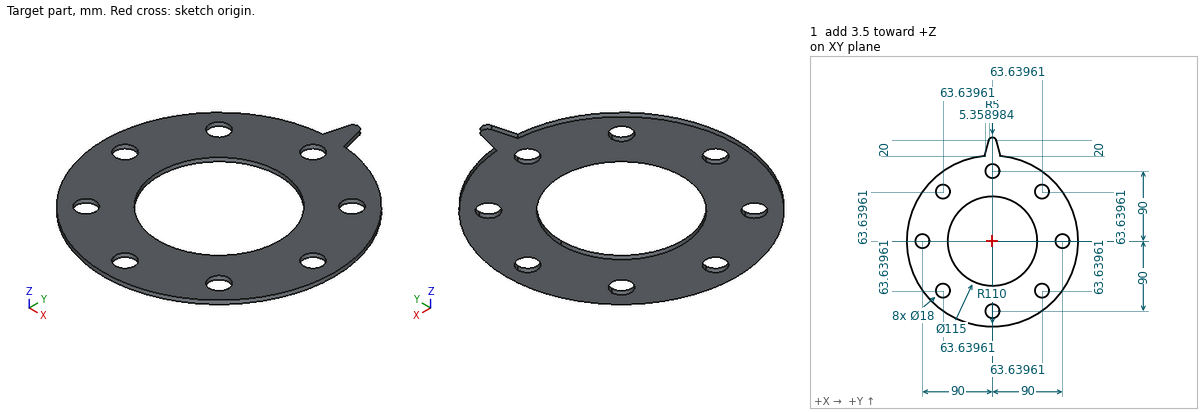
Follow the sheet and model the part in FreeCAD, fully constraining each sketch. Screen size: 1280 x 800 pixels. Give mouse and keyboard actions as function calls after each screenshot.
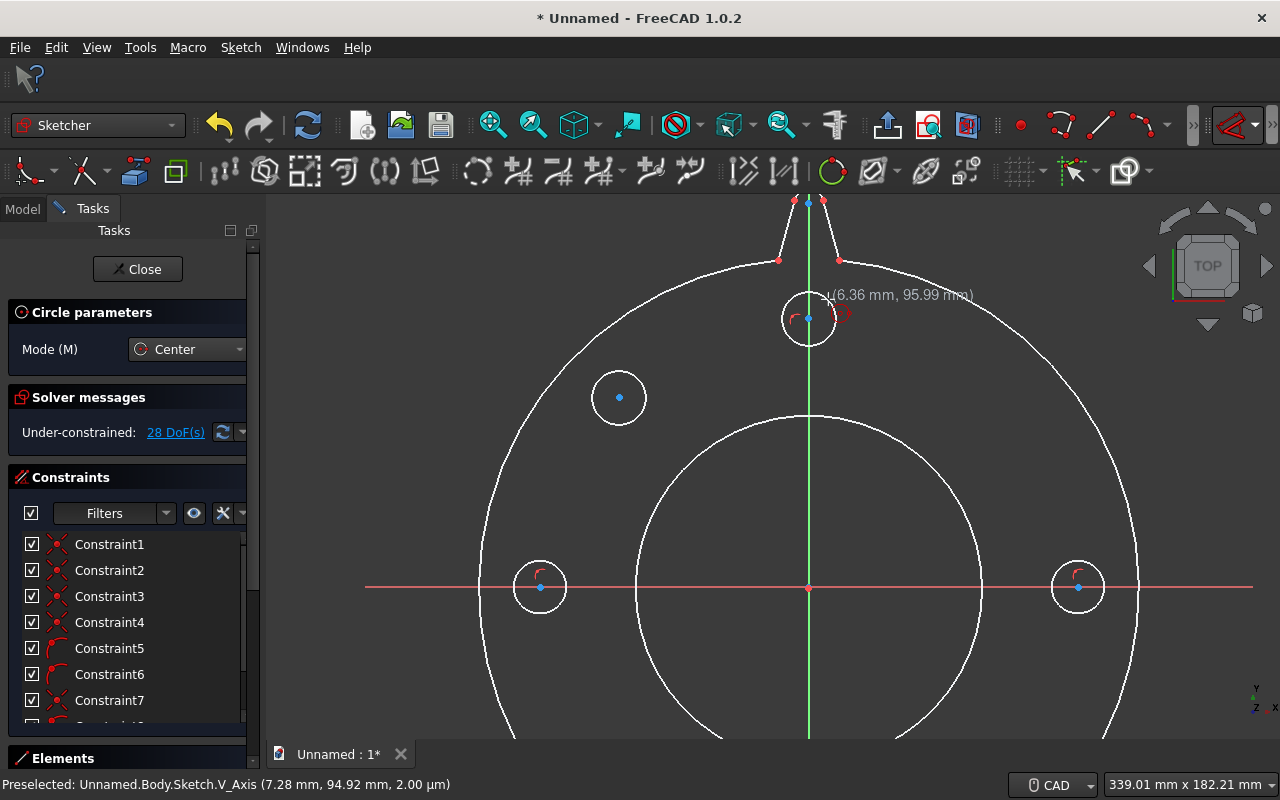
click(999, 397)
click(1018, 378)
key(Escape)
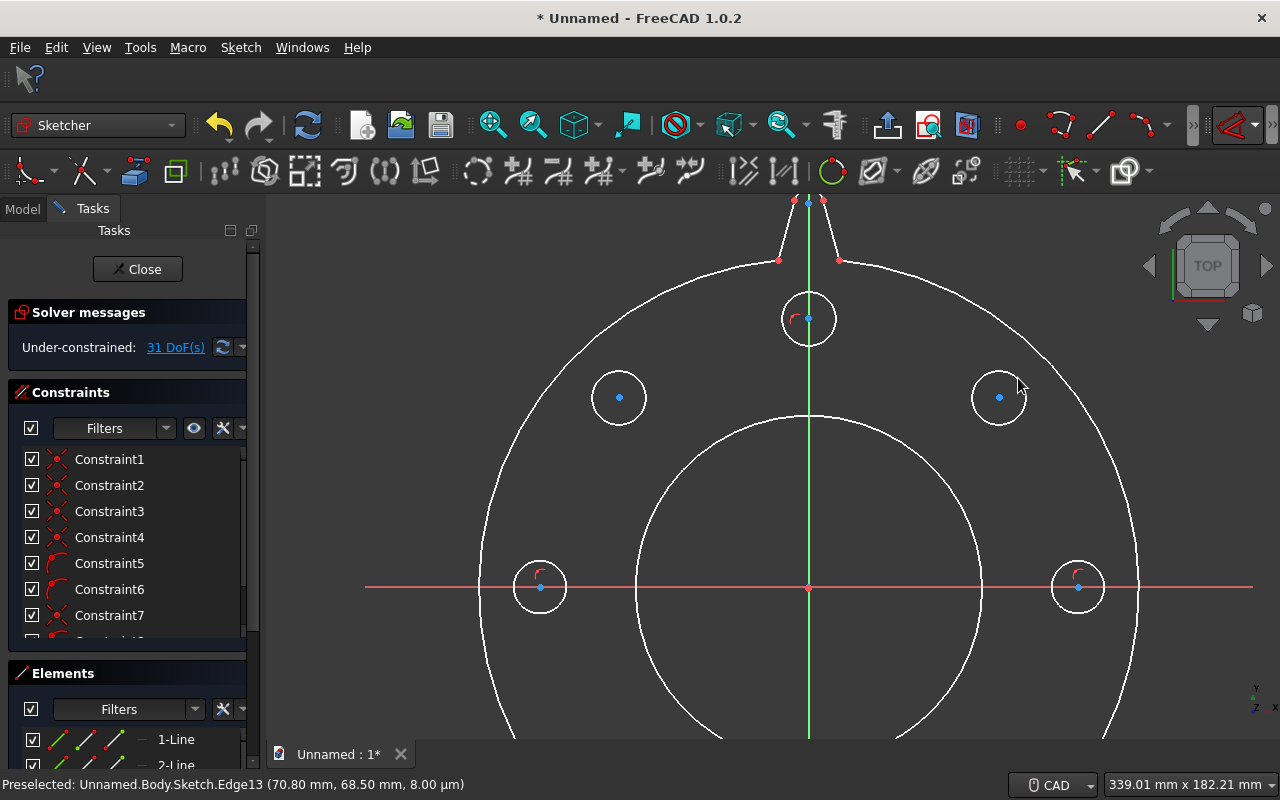
click(783, 242)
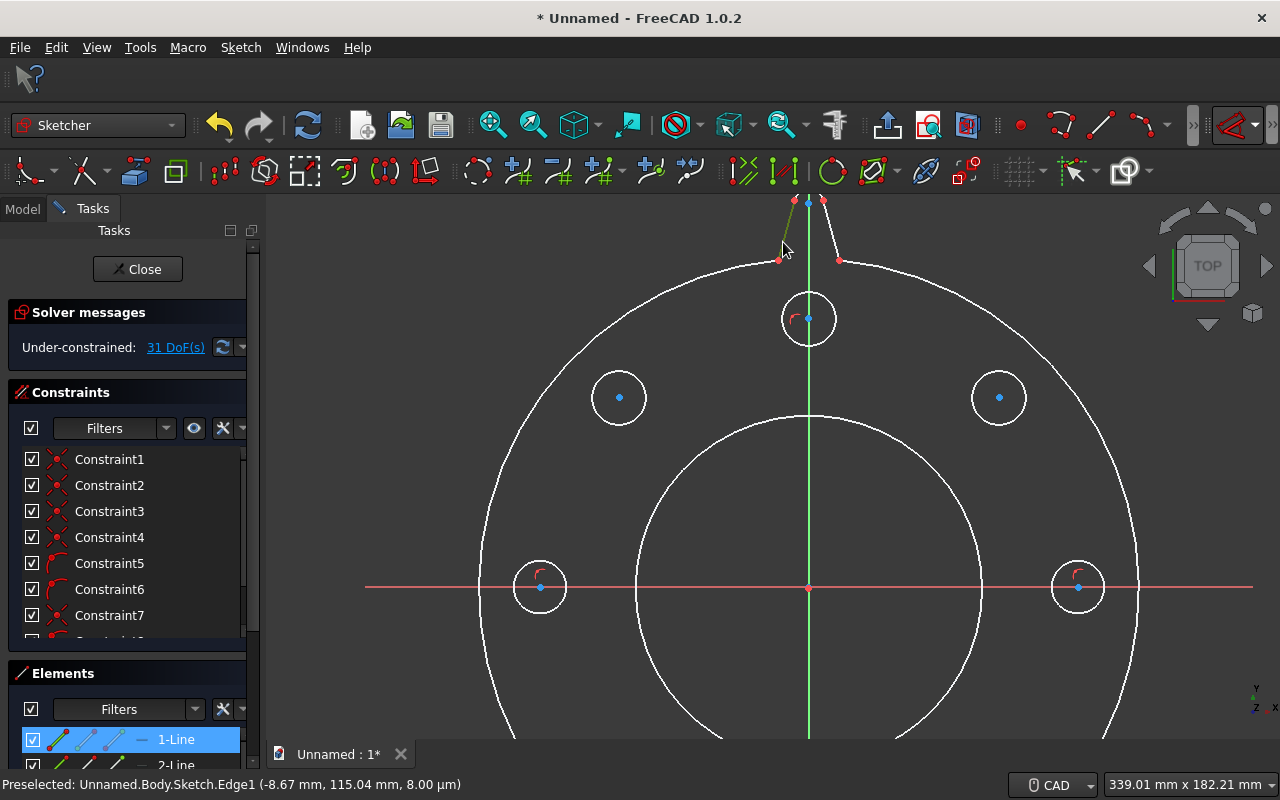
scroll(619, 396, down, 4)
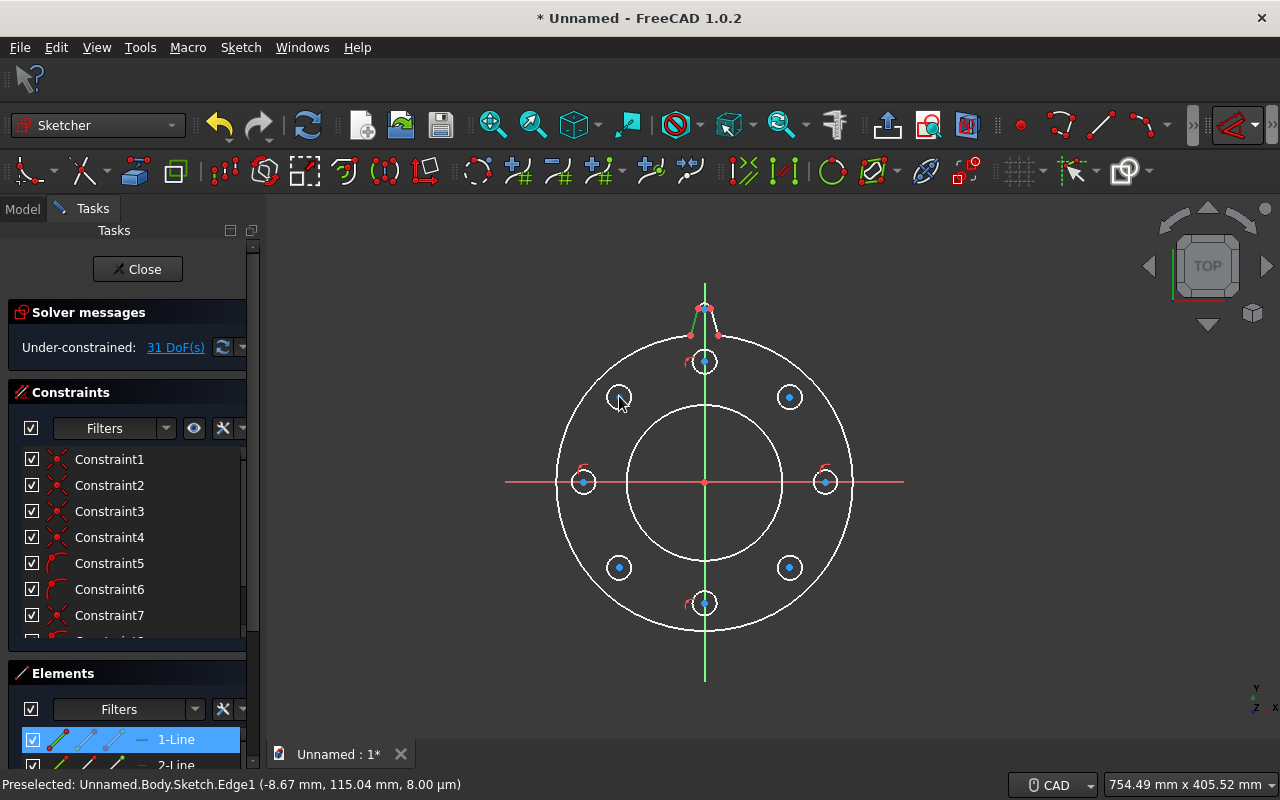
scroll(705, 303, up, 4)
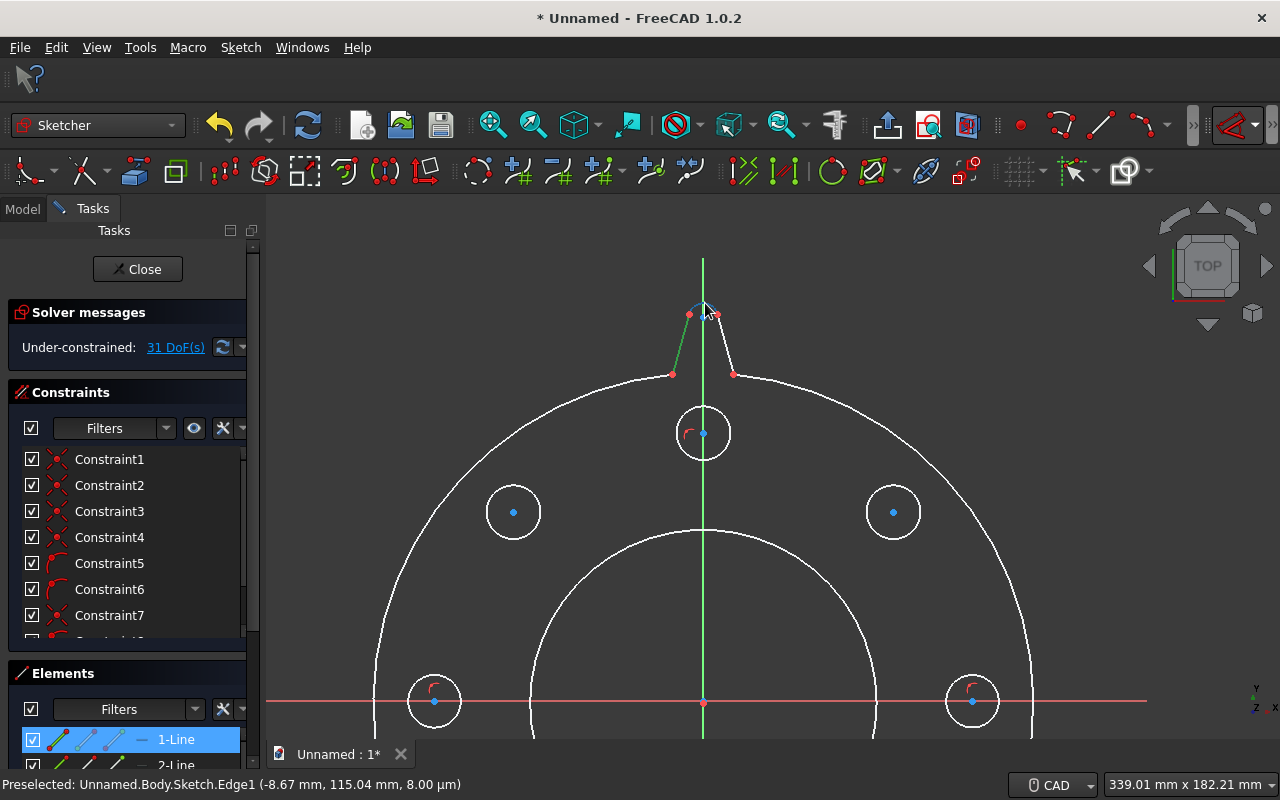
click(703, 303)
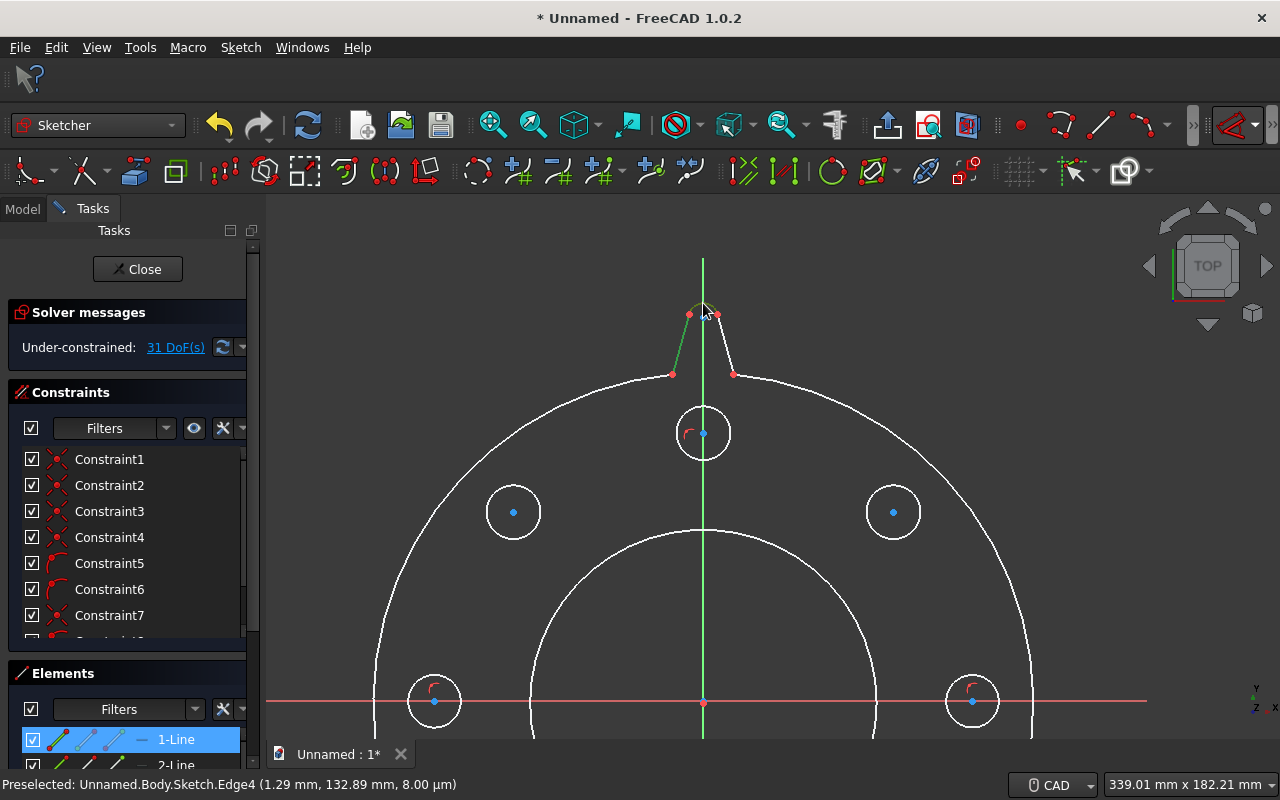
key(t)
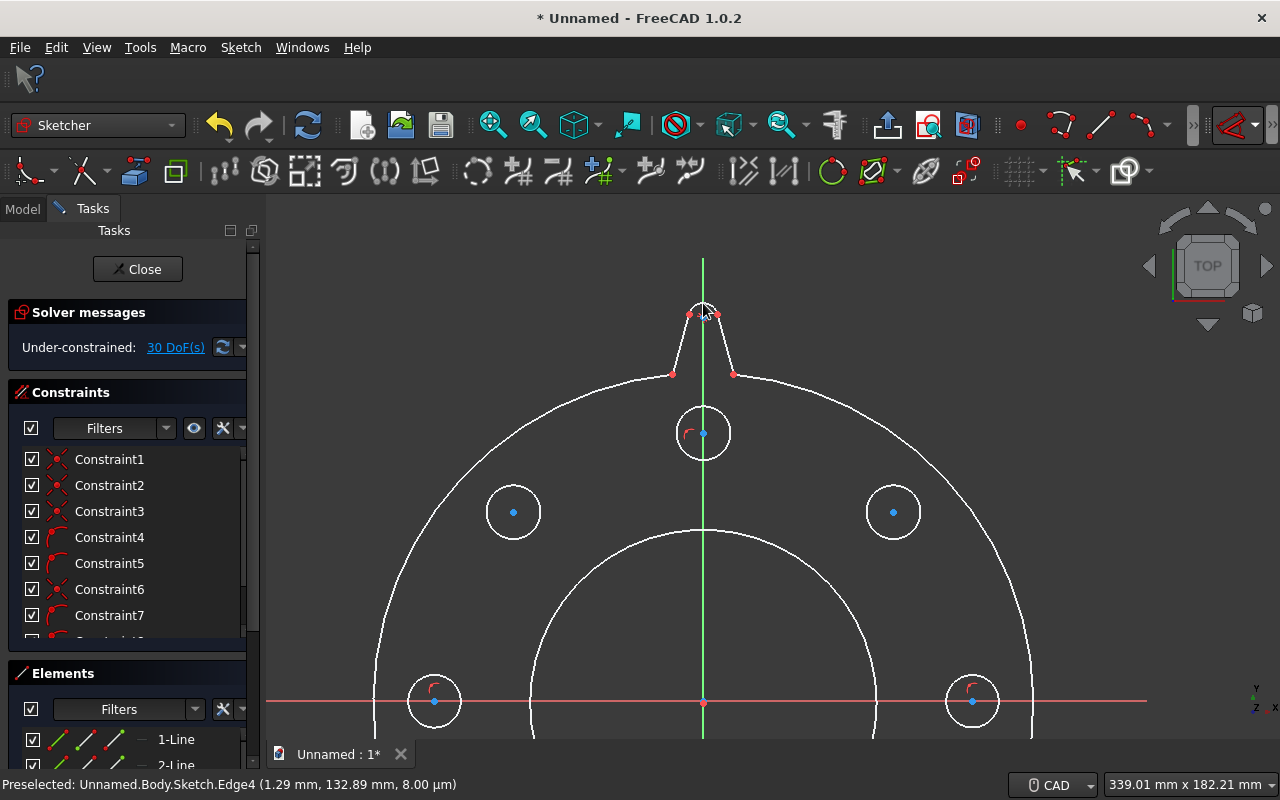
click(729, 357)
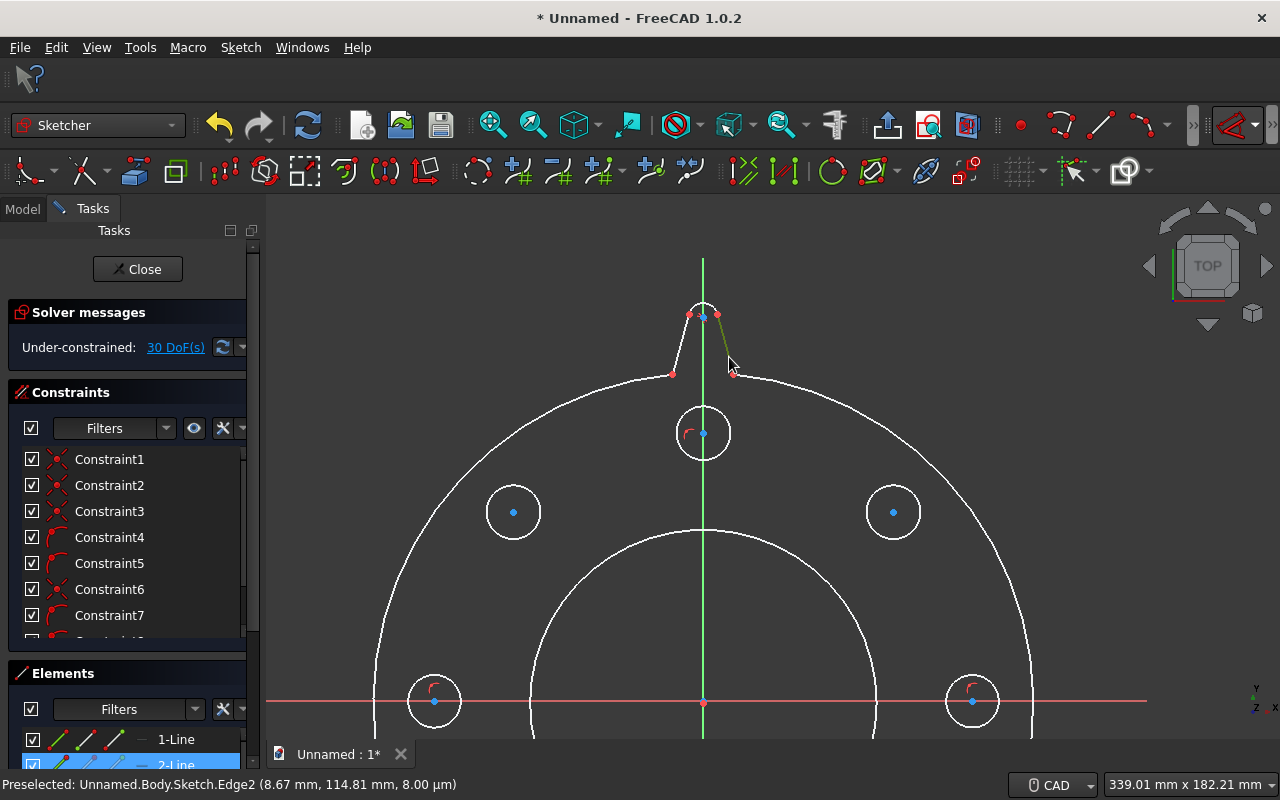
click(704, 303)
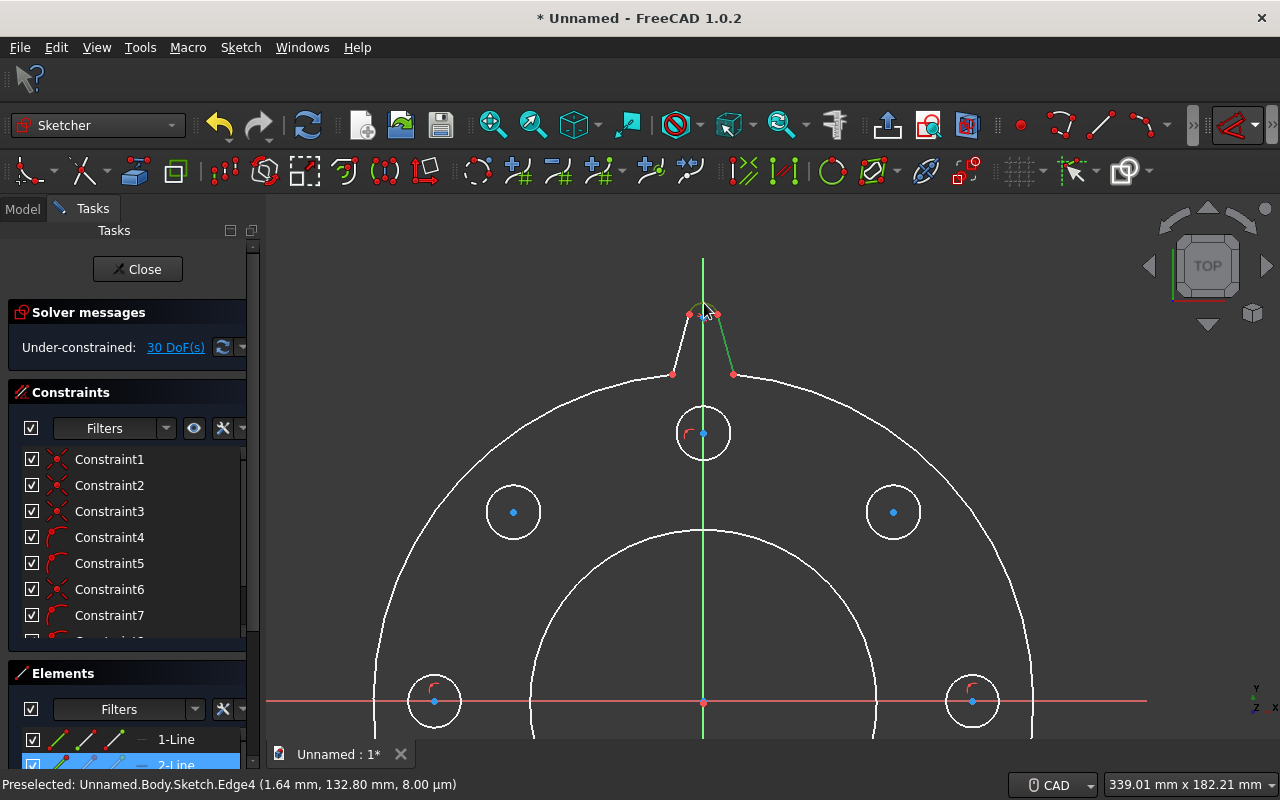
key(t)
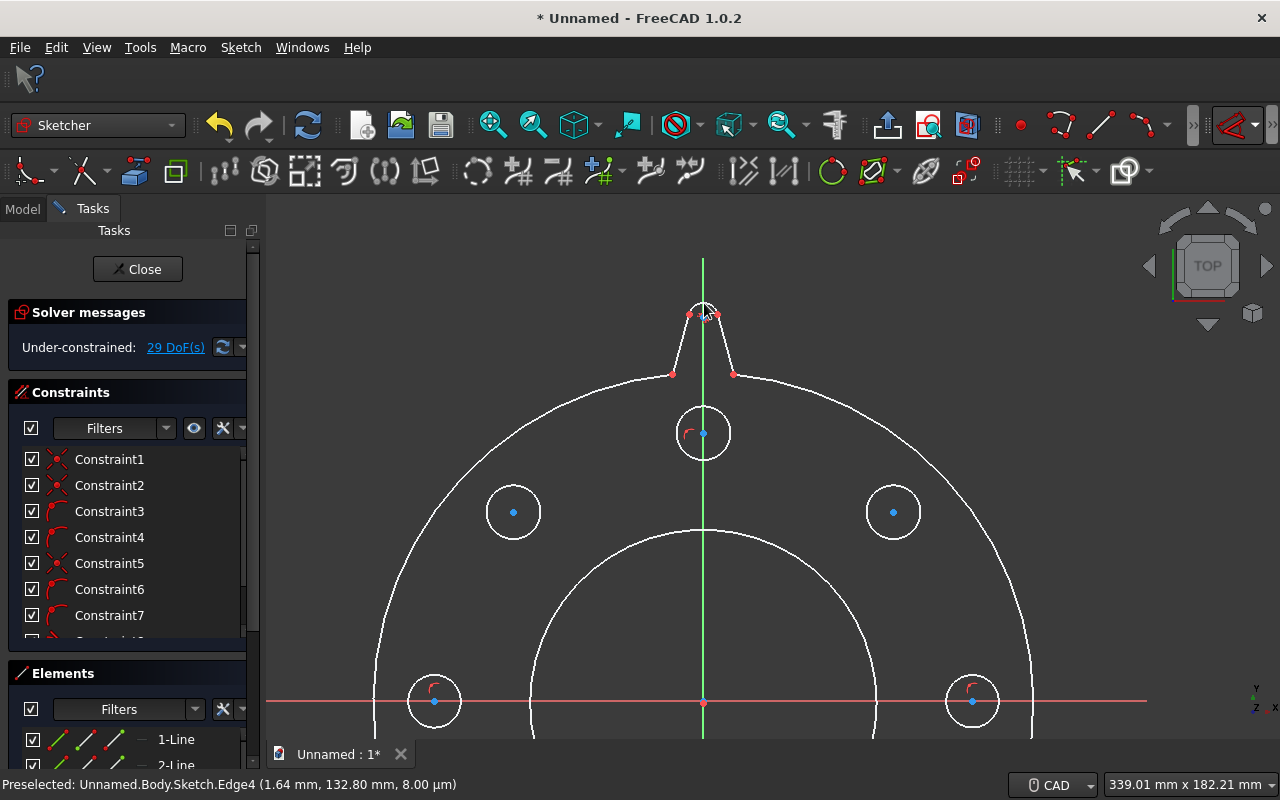
scroll(703, 702, up, 5)